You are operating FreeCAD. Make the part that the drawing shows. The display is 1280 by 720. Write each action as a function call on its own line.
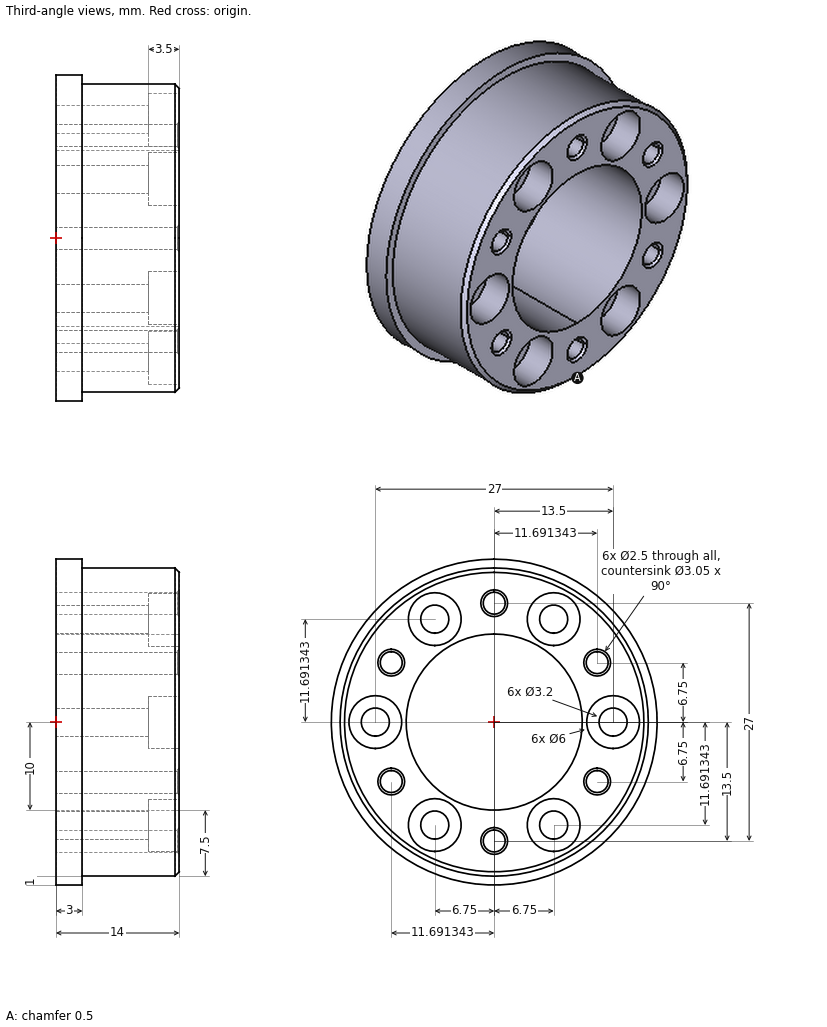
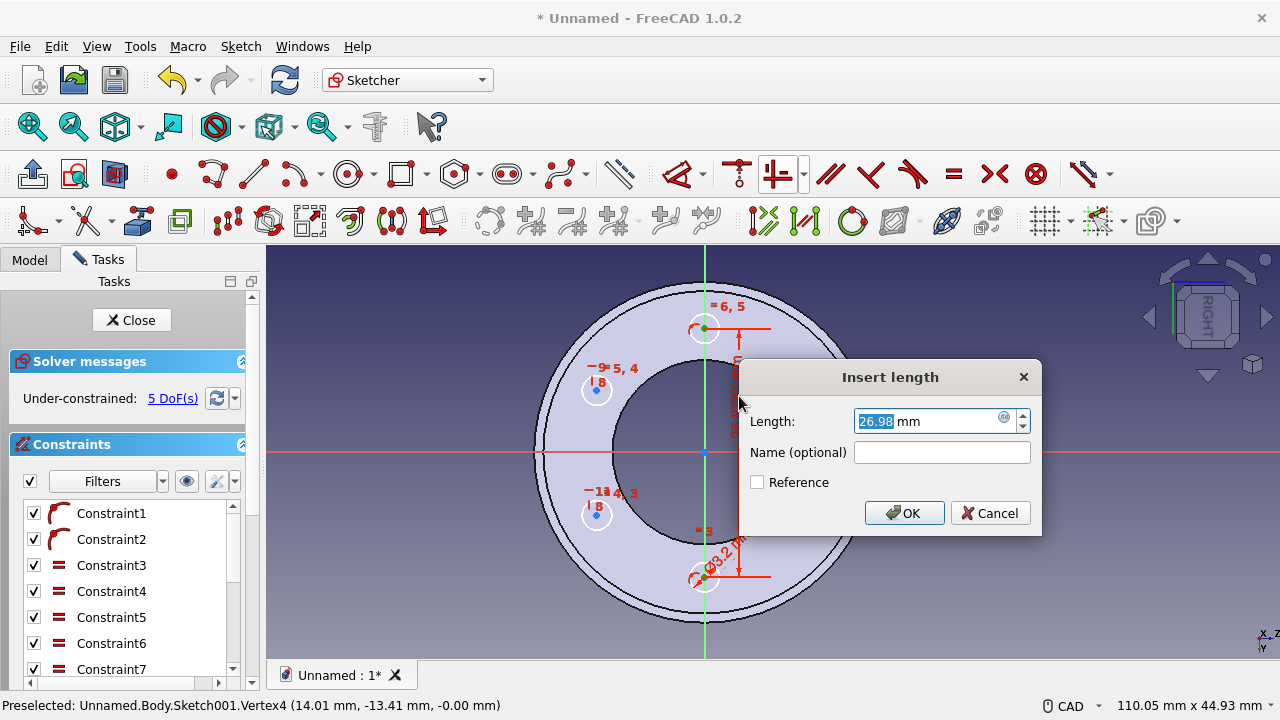
text(27)
key(Return)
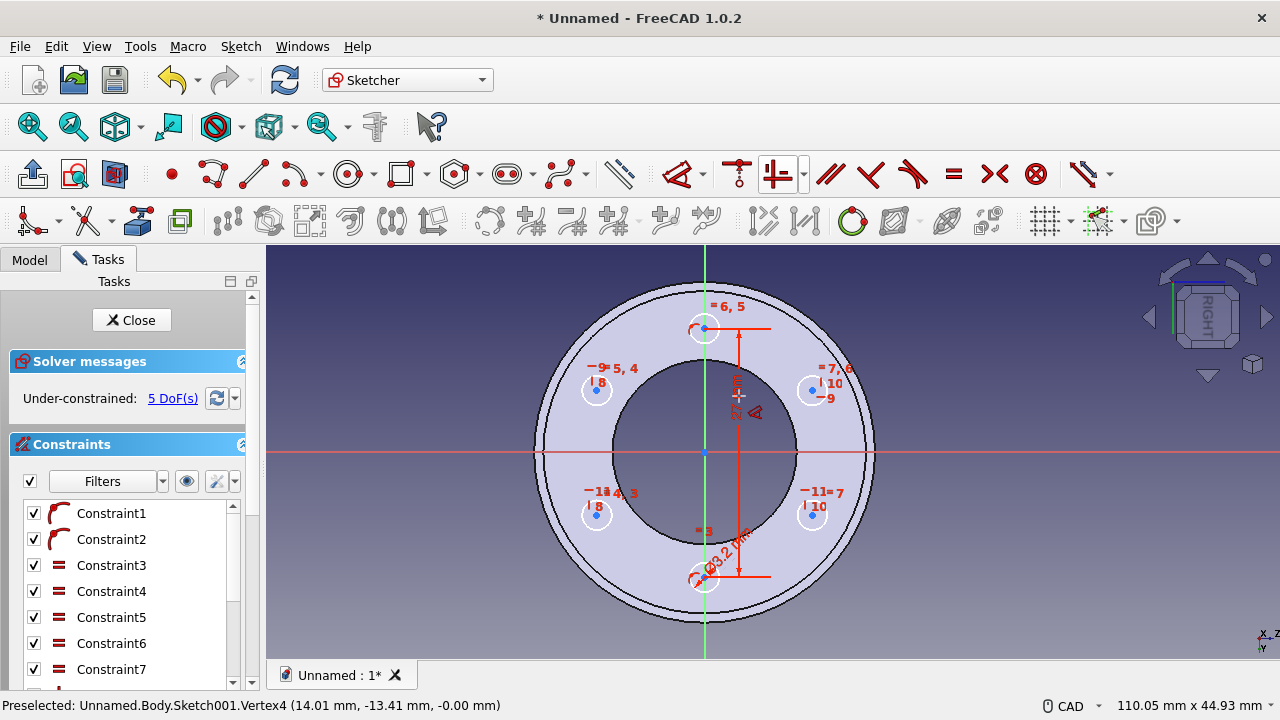
click(705, 577)
click(739, 515)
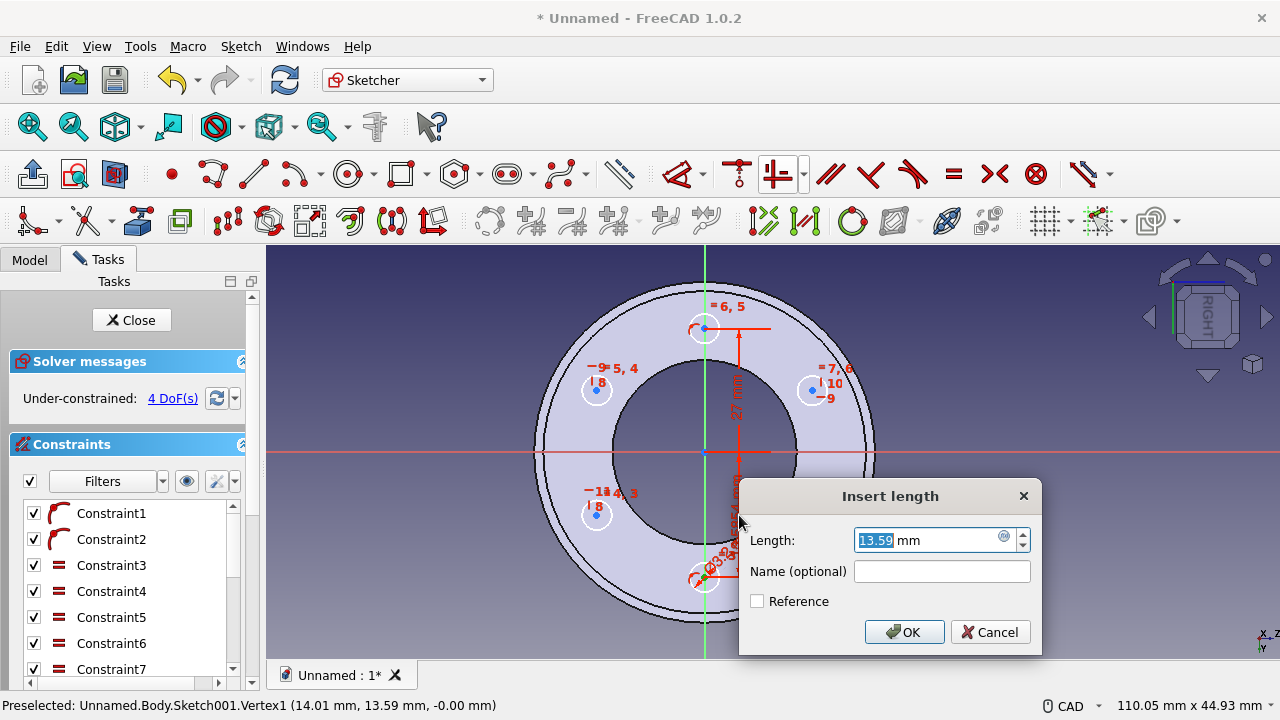
text(13.5)
key(Return)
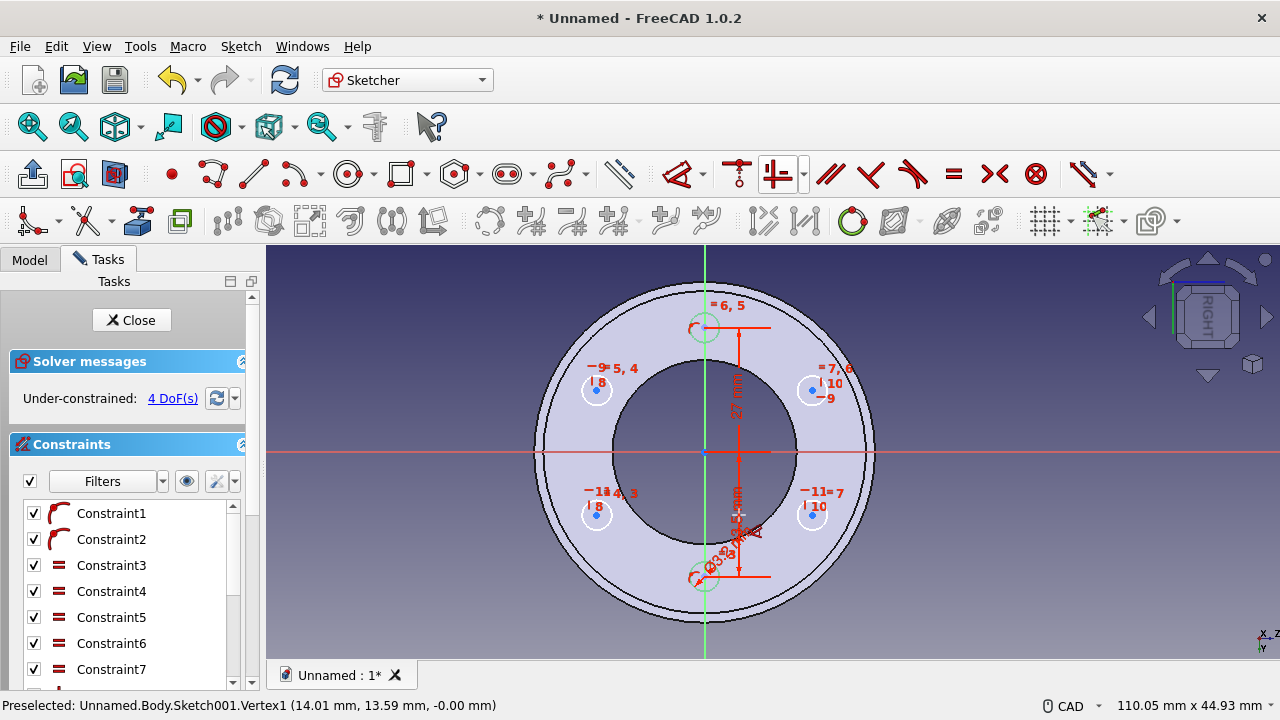
click(597, 515)
click(563, 484)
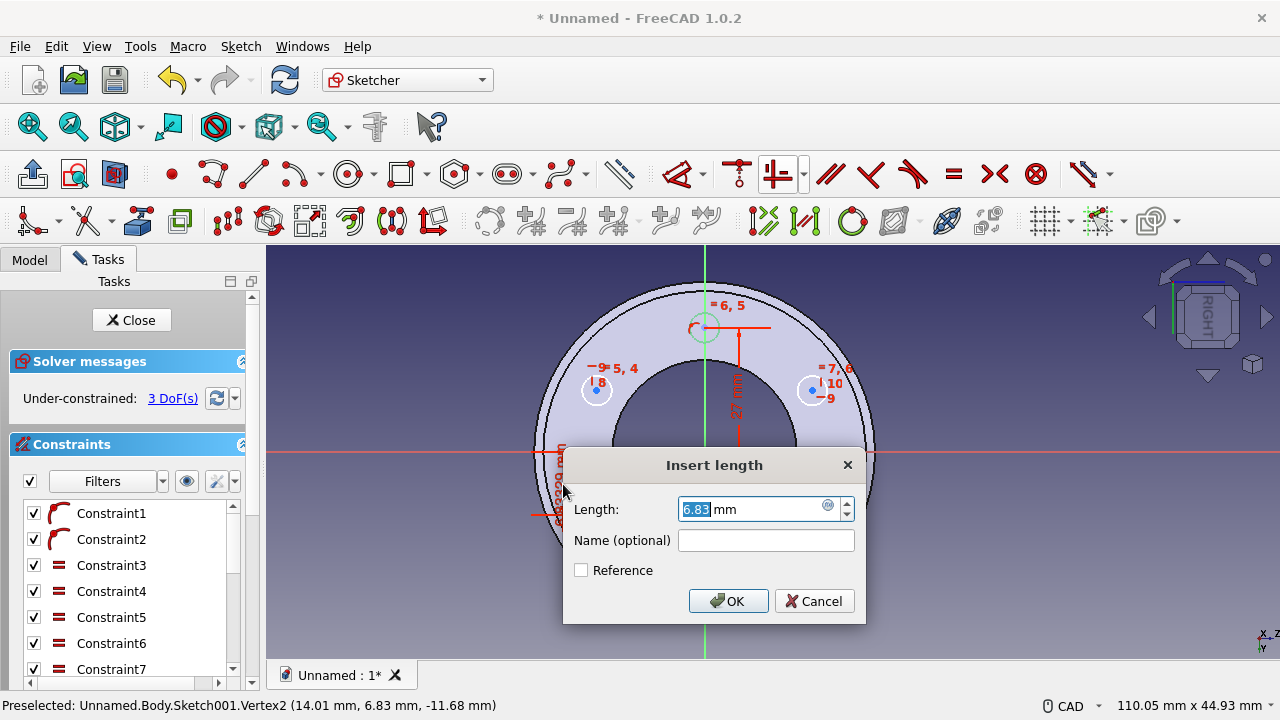
text(6.75)
key(Return)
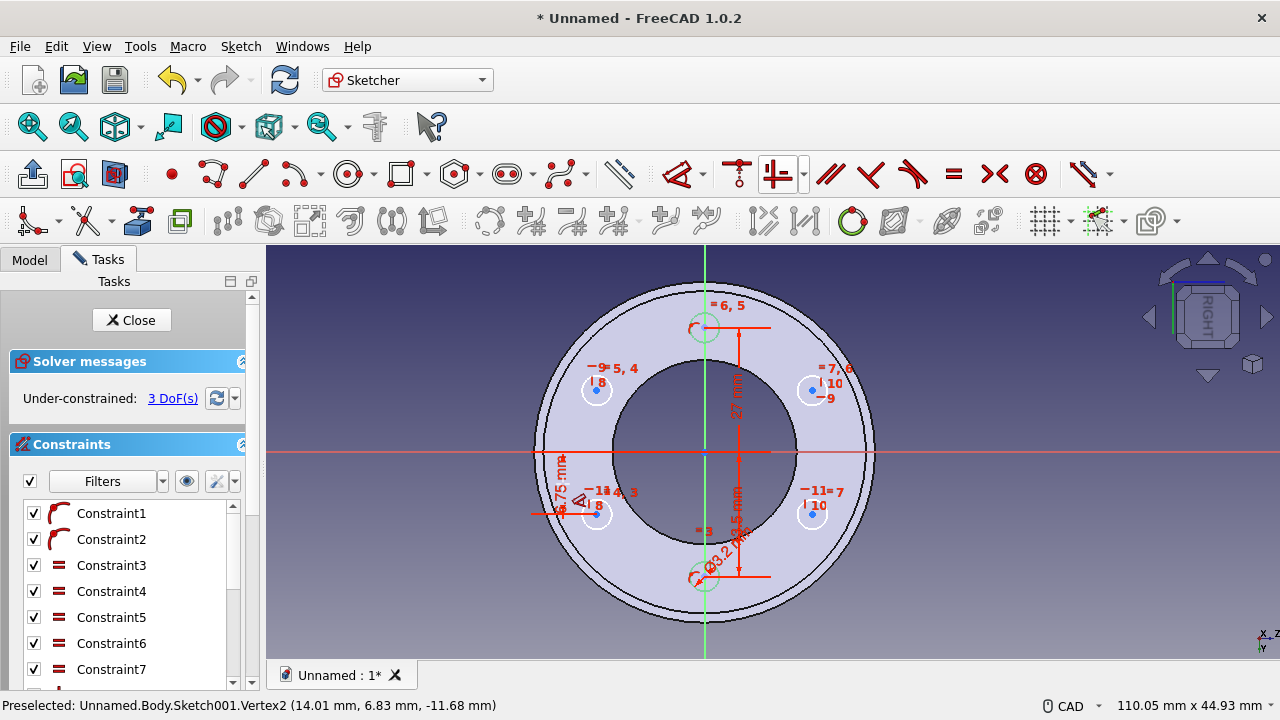
click(597, 391)
click(563, 421)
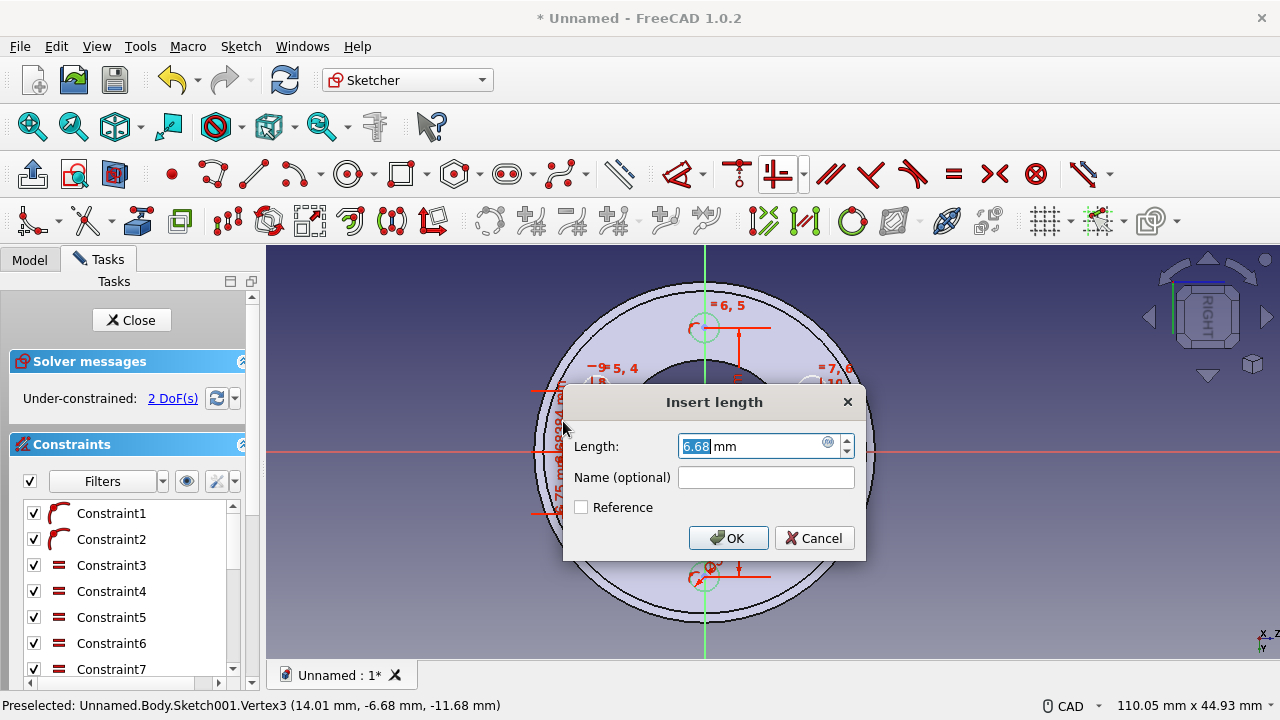
text(6.75)
key(Return)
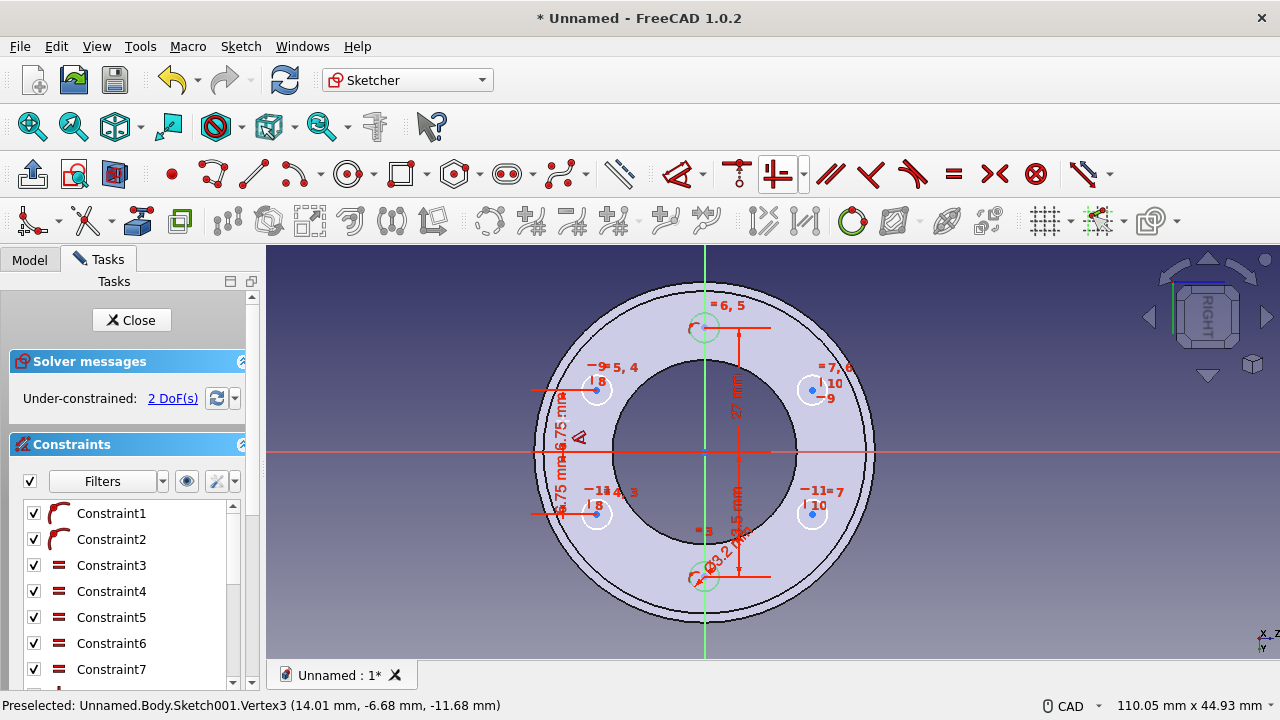
click(597, 514)
click(651, 548)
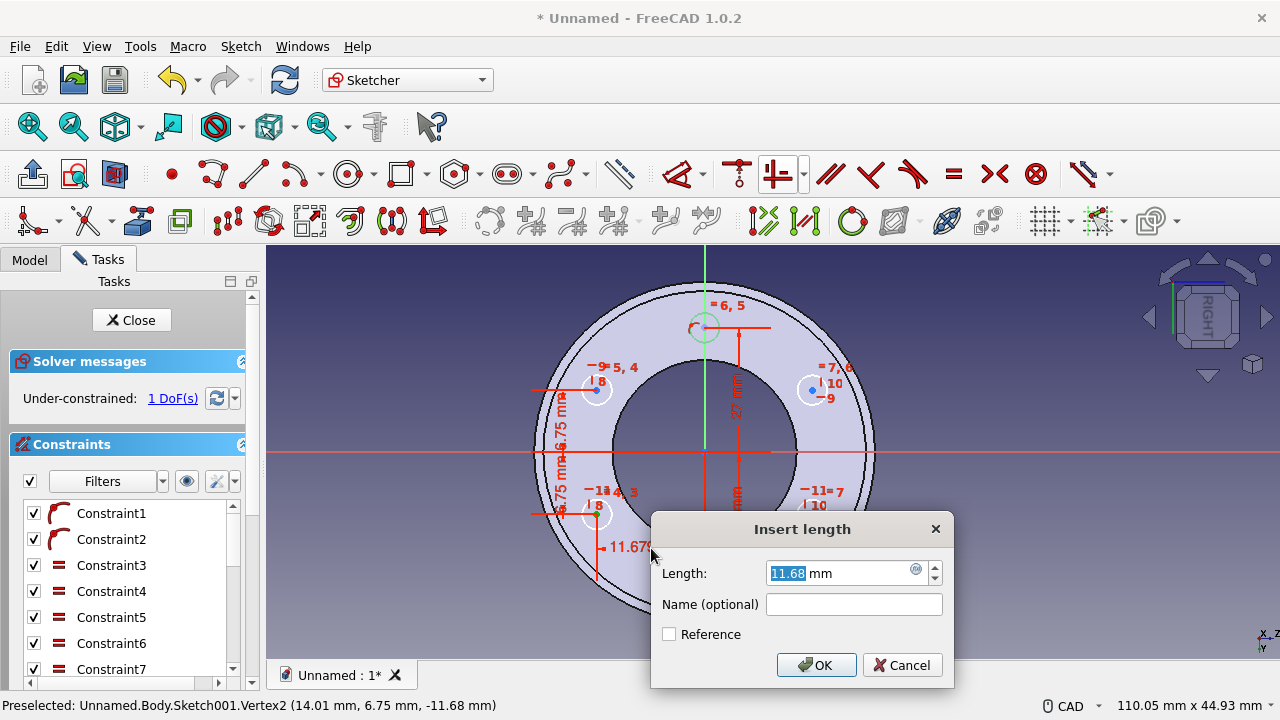
text(11.691343)
key(Return)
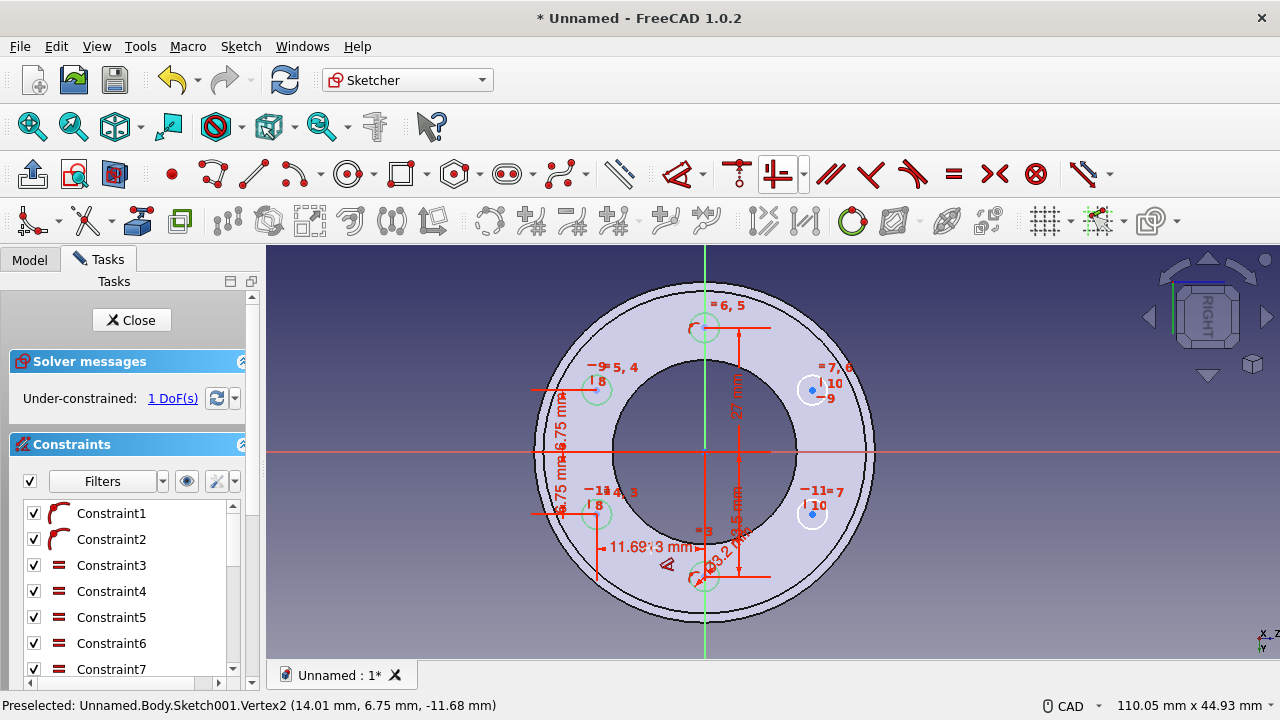
click(812, 390)
click(758, 356)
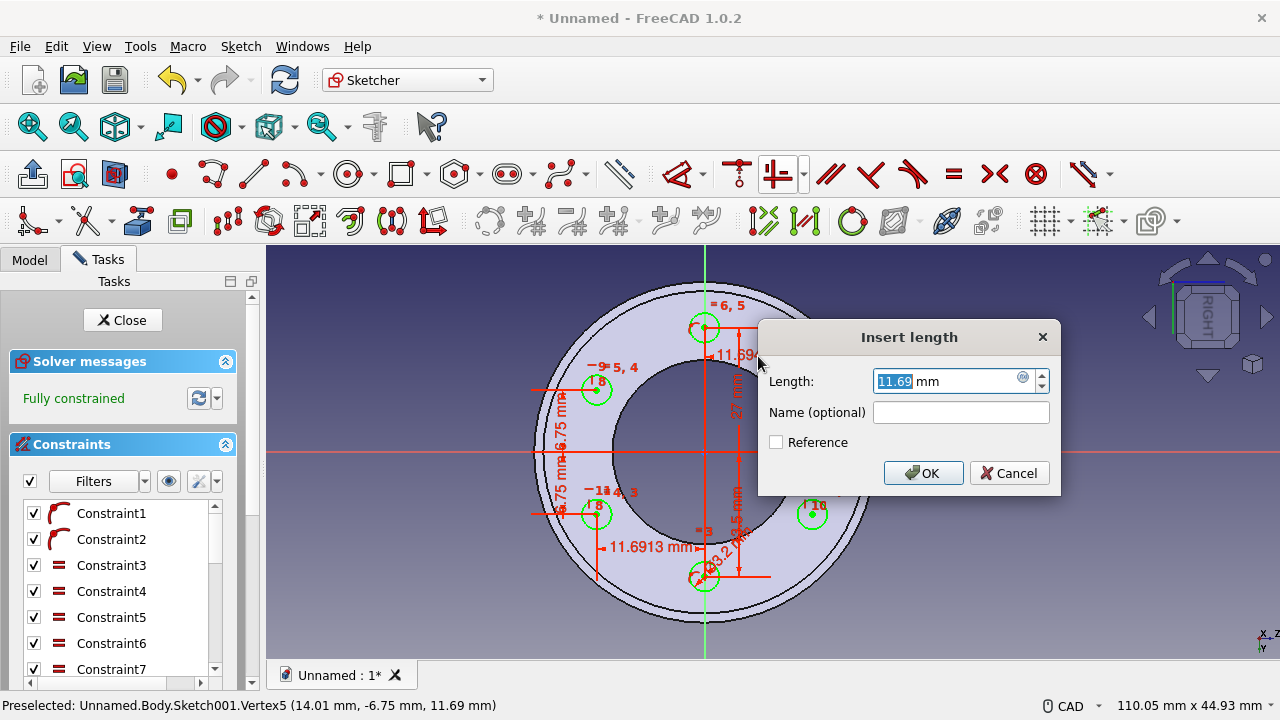
text(11.691343)
key(Return)
key(Escape)